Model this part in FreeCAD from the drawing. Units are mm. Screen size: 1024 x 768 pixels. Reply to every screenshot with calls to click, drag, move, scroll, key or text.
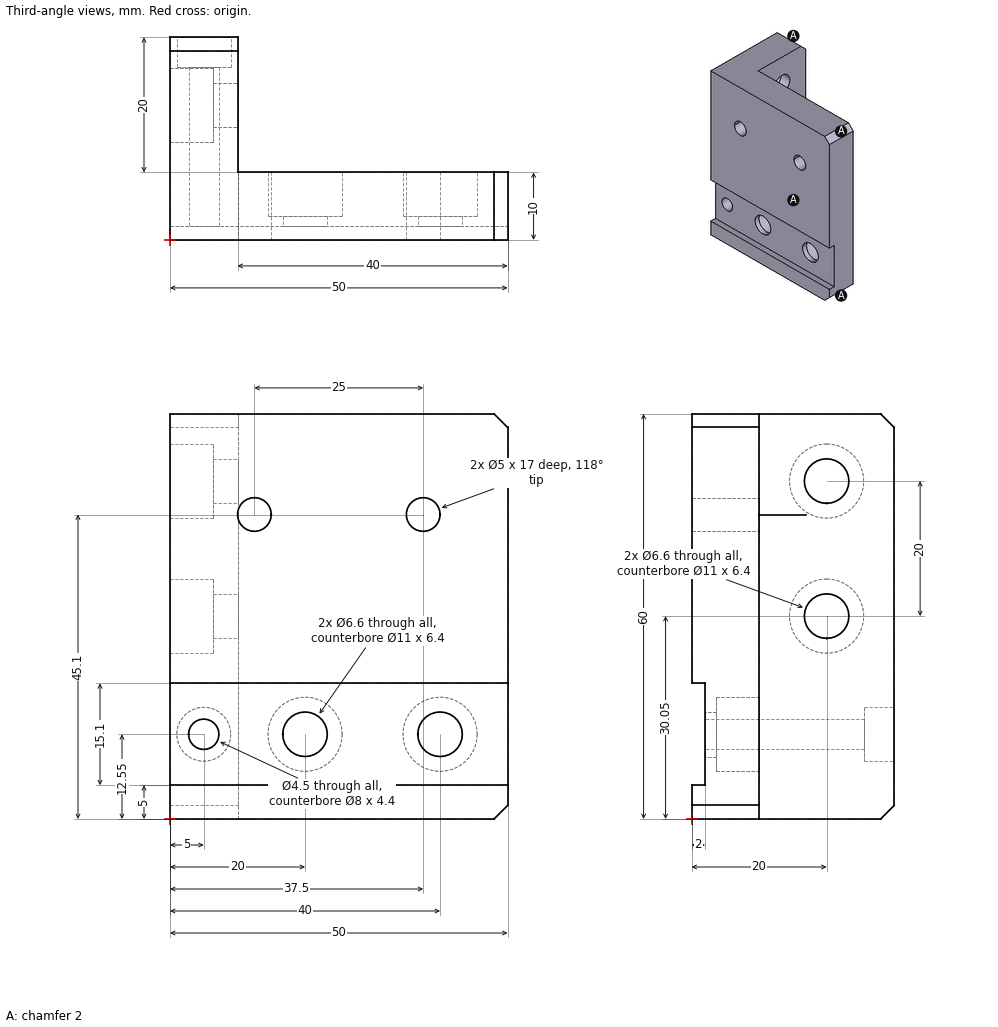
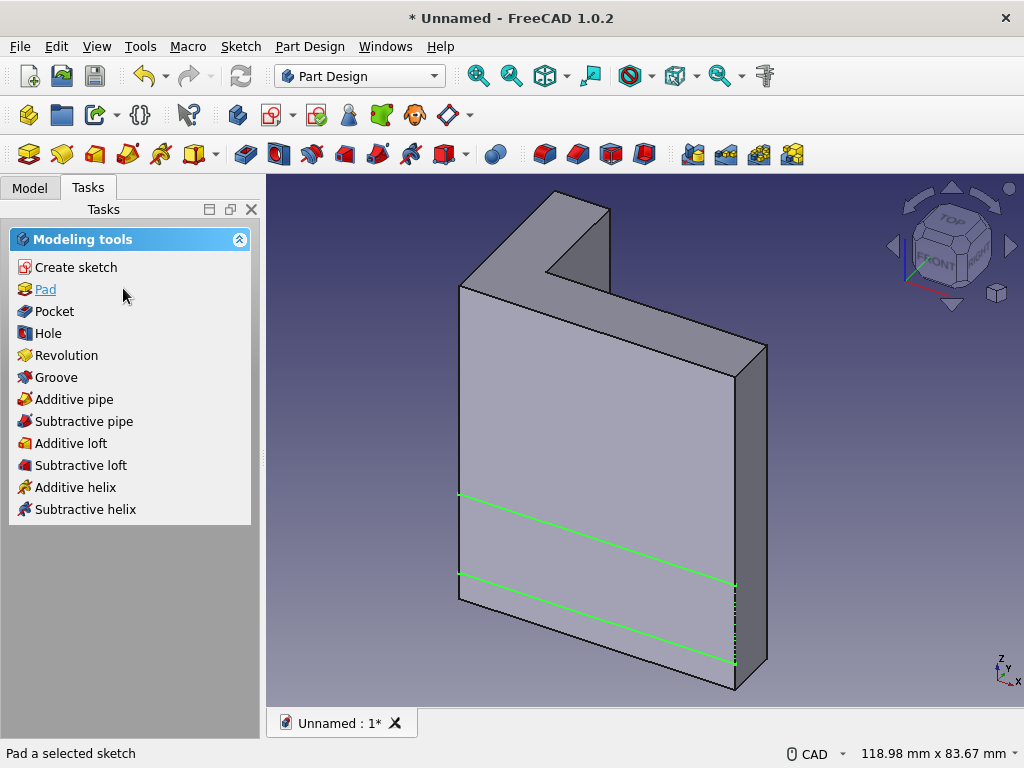
click(246, 154)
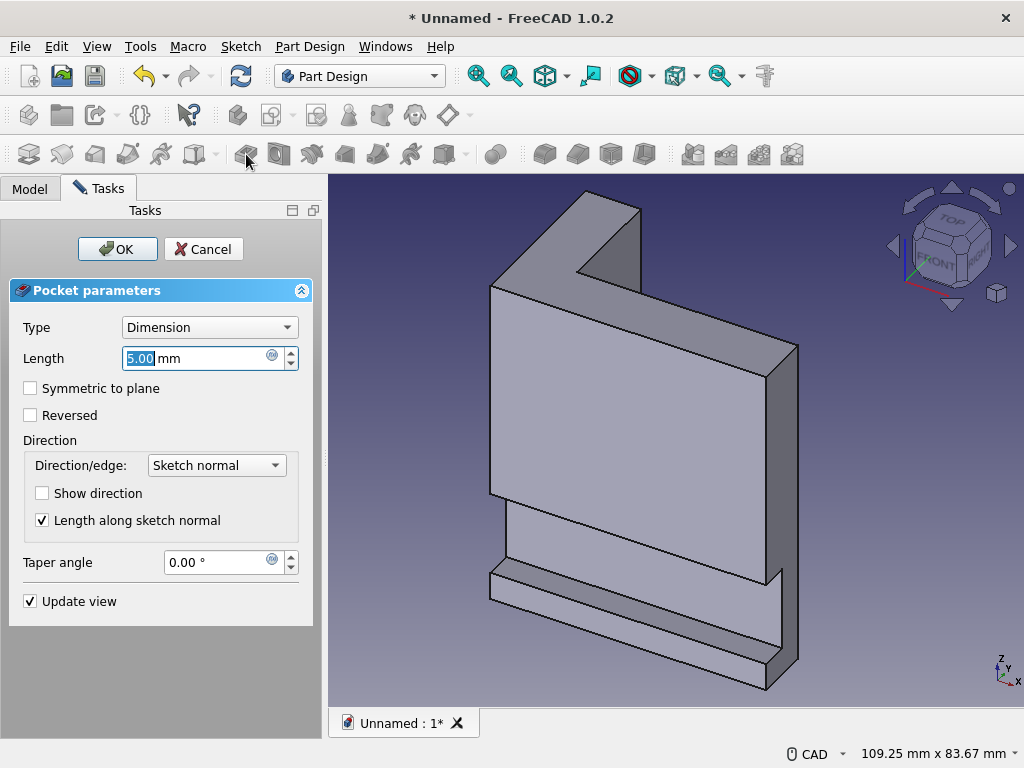
text(2)
key(Tab)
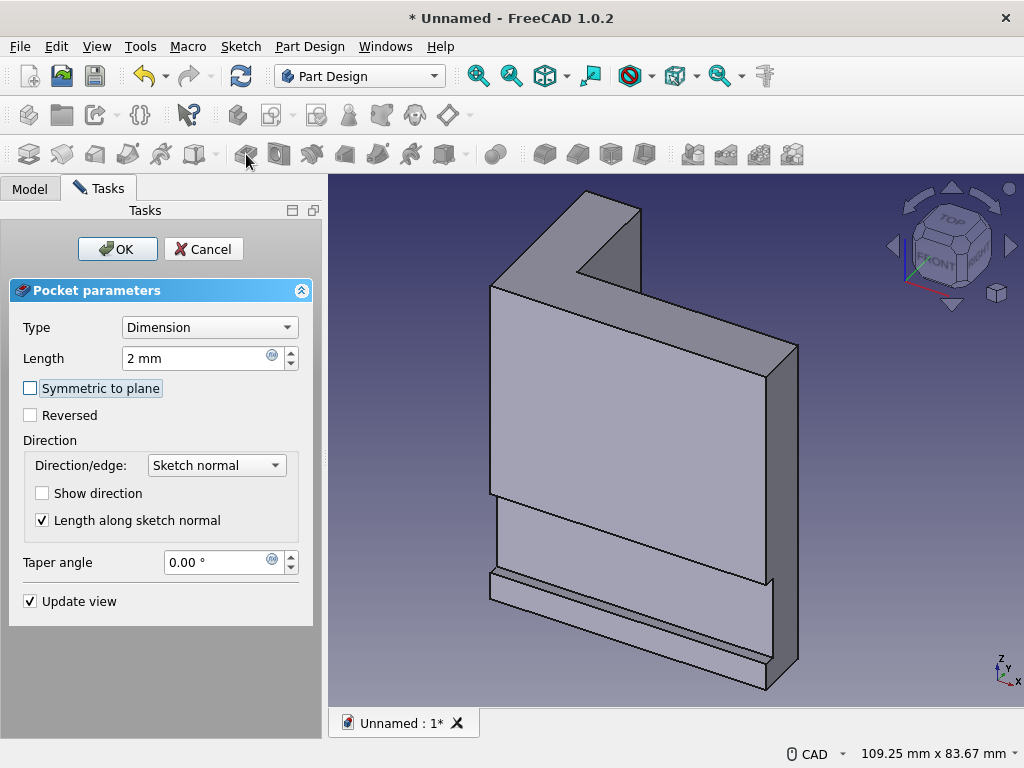
click(118, 249)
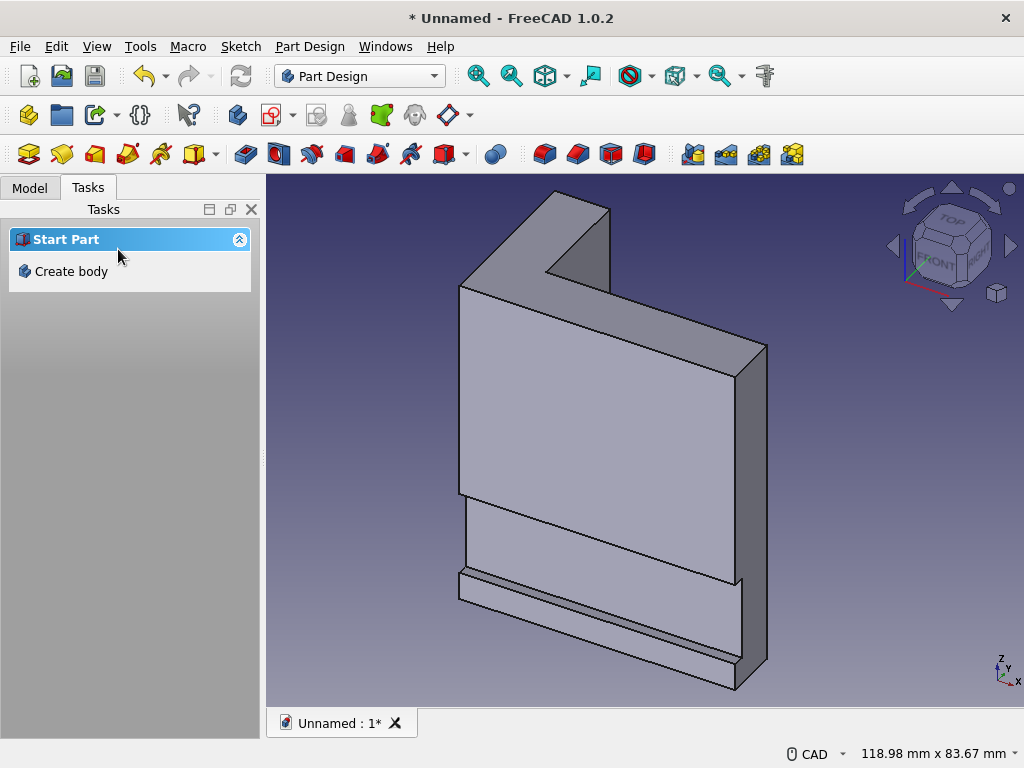
key(4)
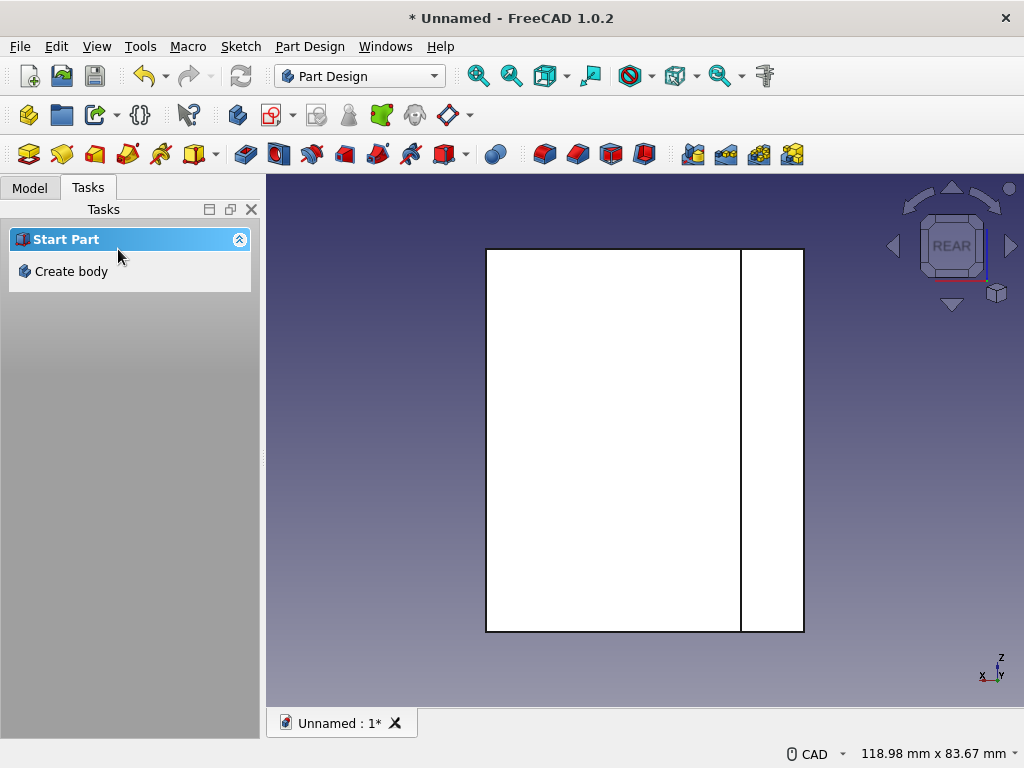
click(772, 330)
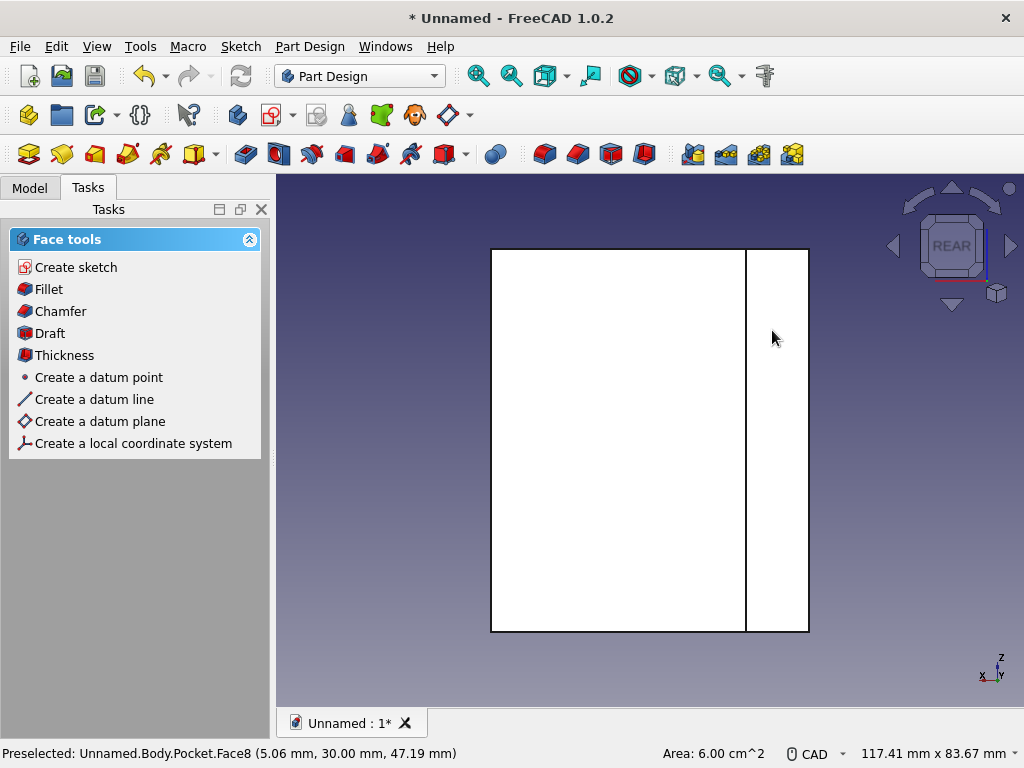
click(270, 116)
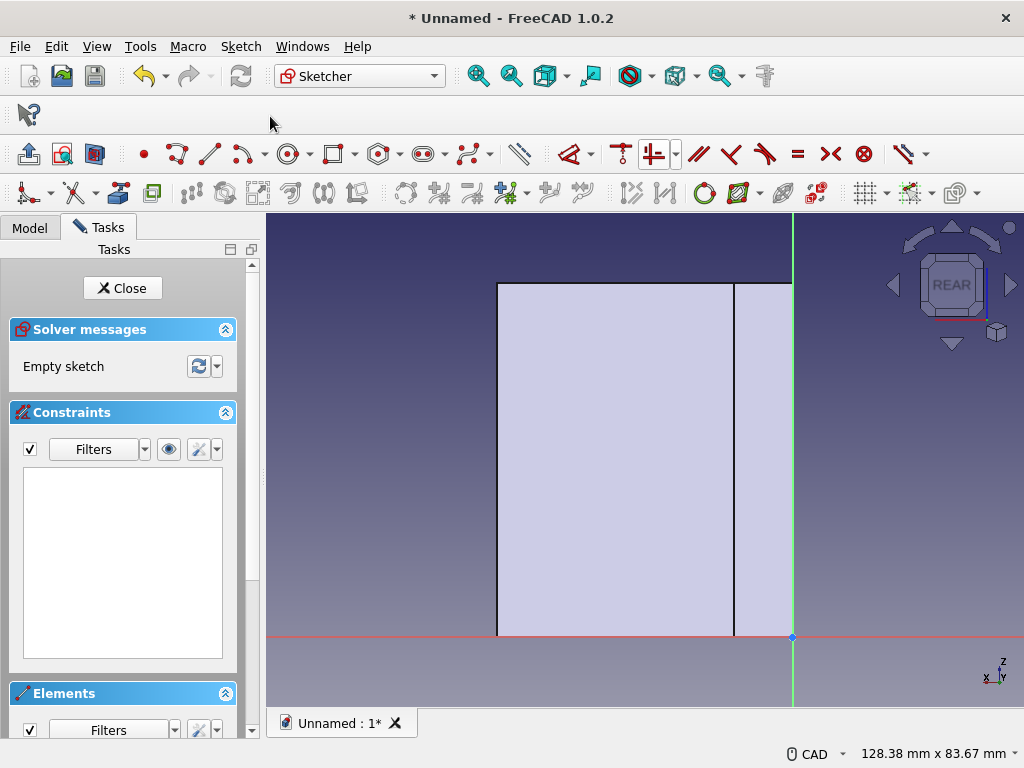
scroll(782, 573, up, 12)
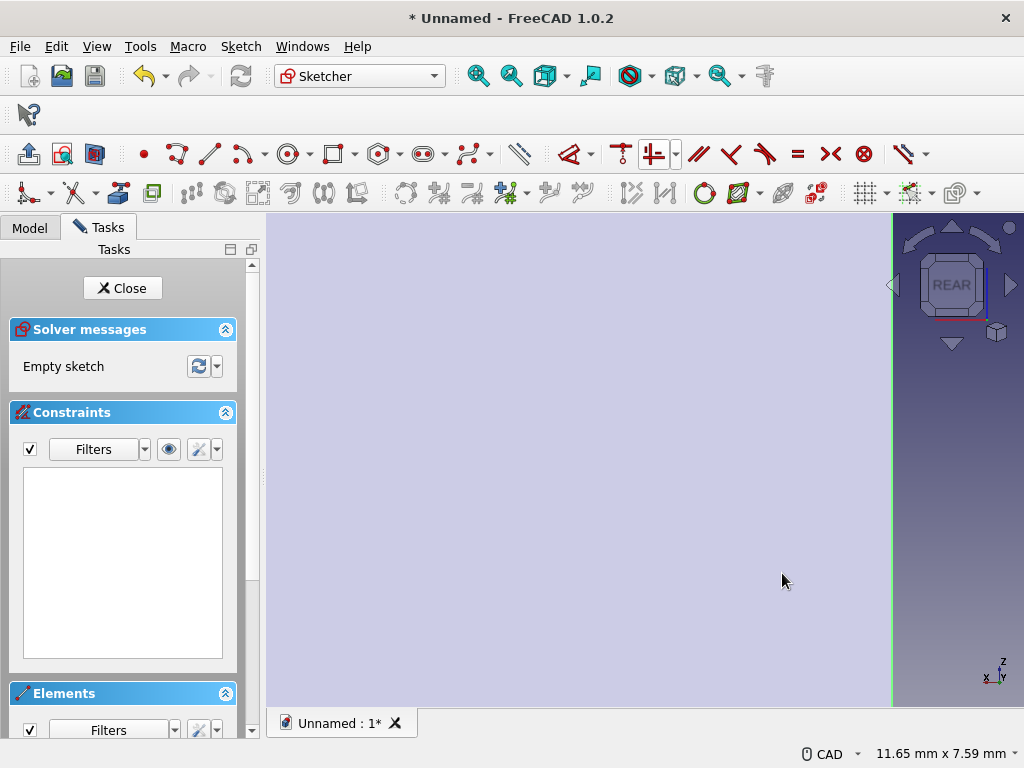
click(288, 154)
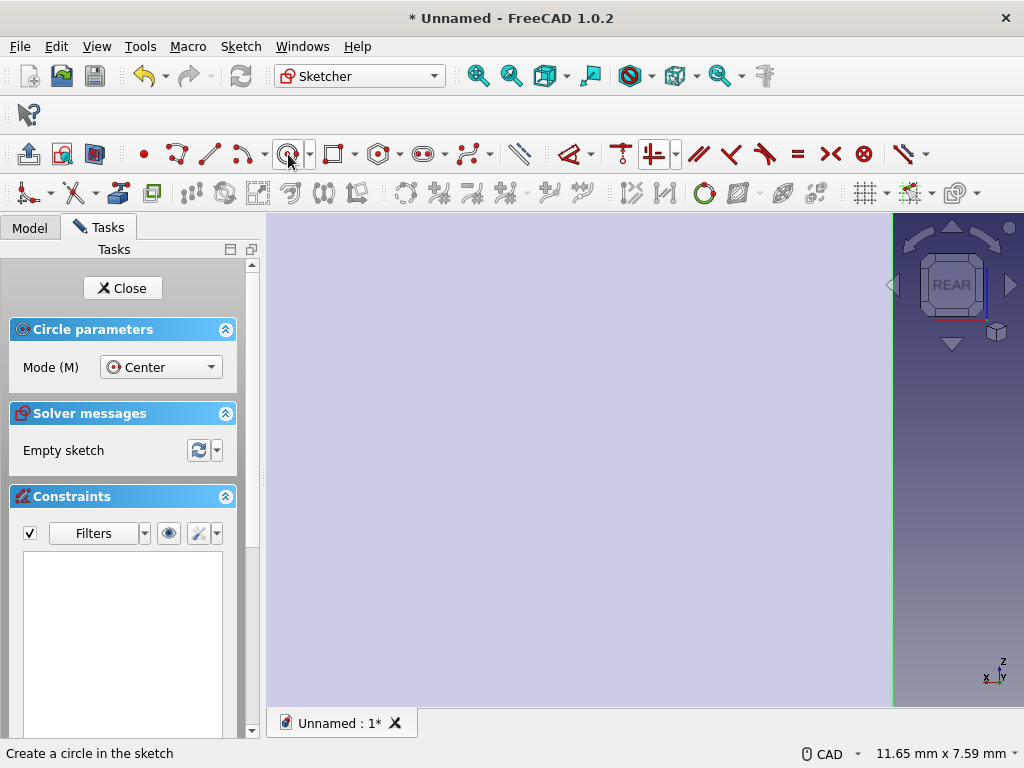
click(567, 456)
click(670, 352)
key(Escape)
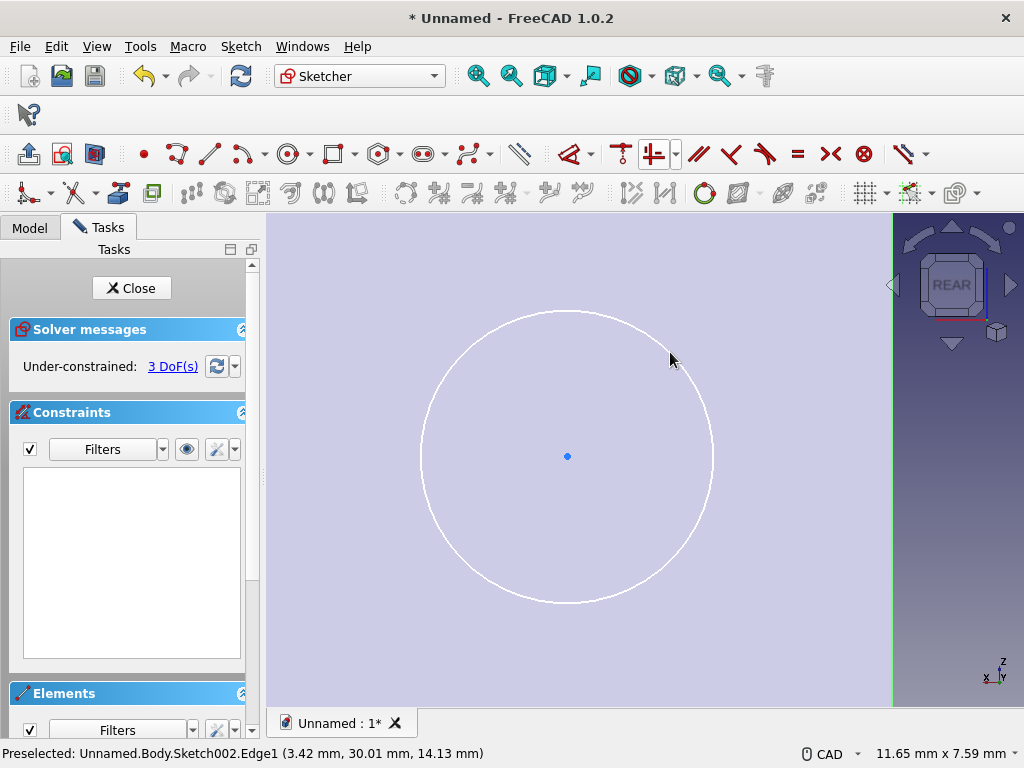
key(d)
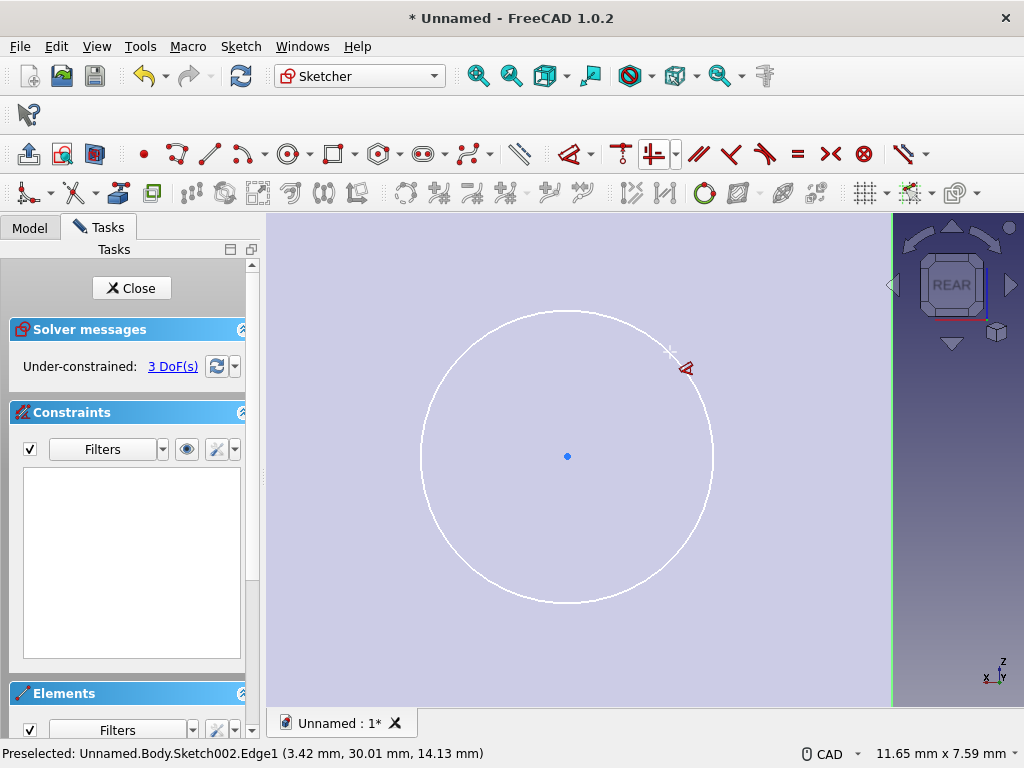
click(670, 353)
click(693, 330)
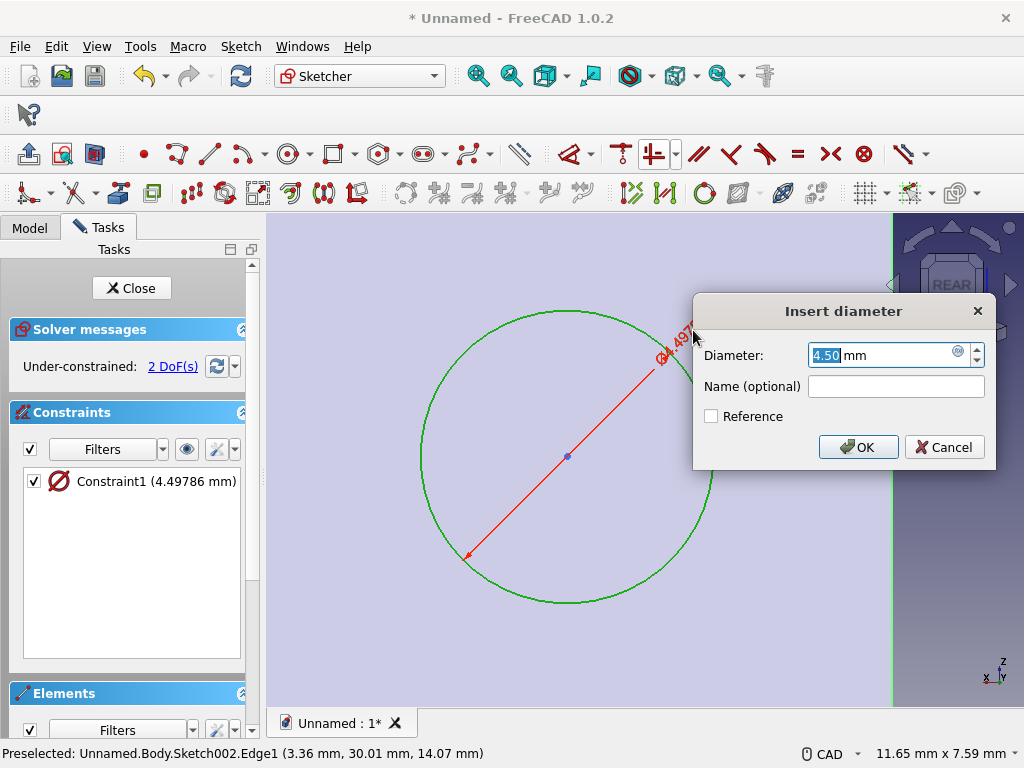
text(4.5)
key(Return)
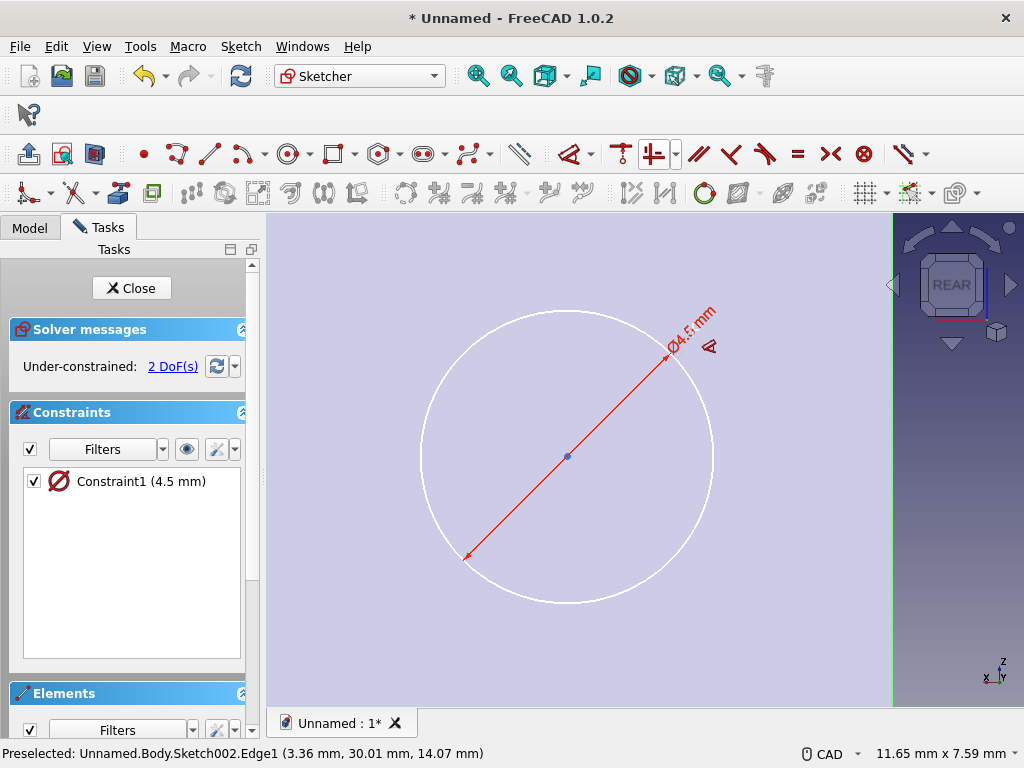
click(567, 457)
click(646, 423)